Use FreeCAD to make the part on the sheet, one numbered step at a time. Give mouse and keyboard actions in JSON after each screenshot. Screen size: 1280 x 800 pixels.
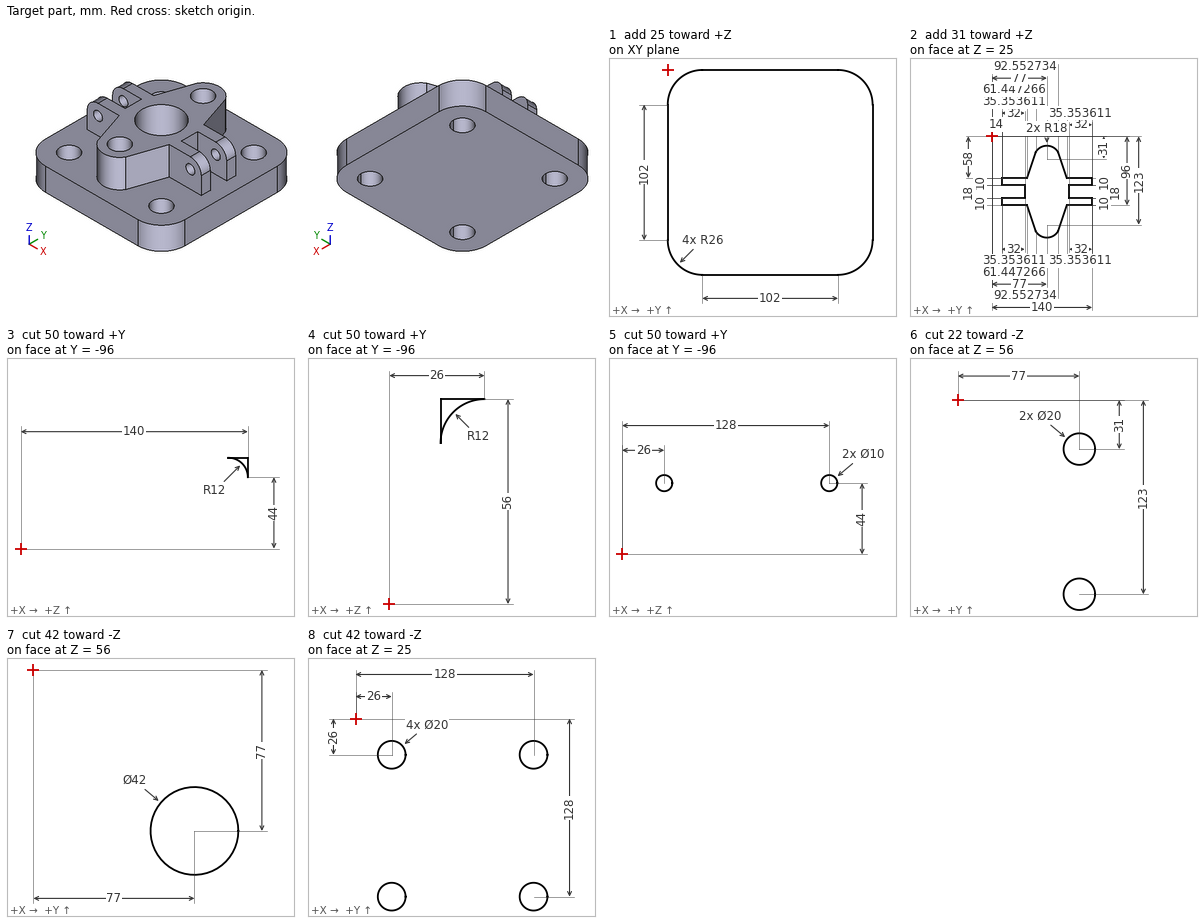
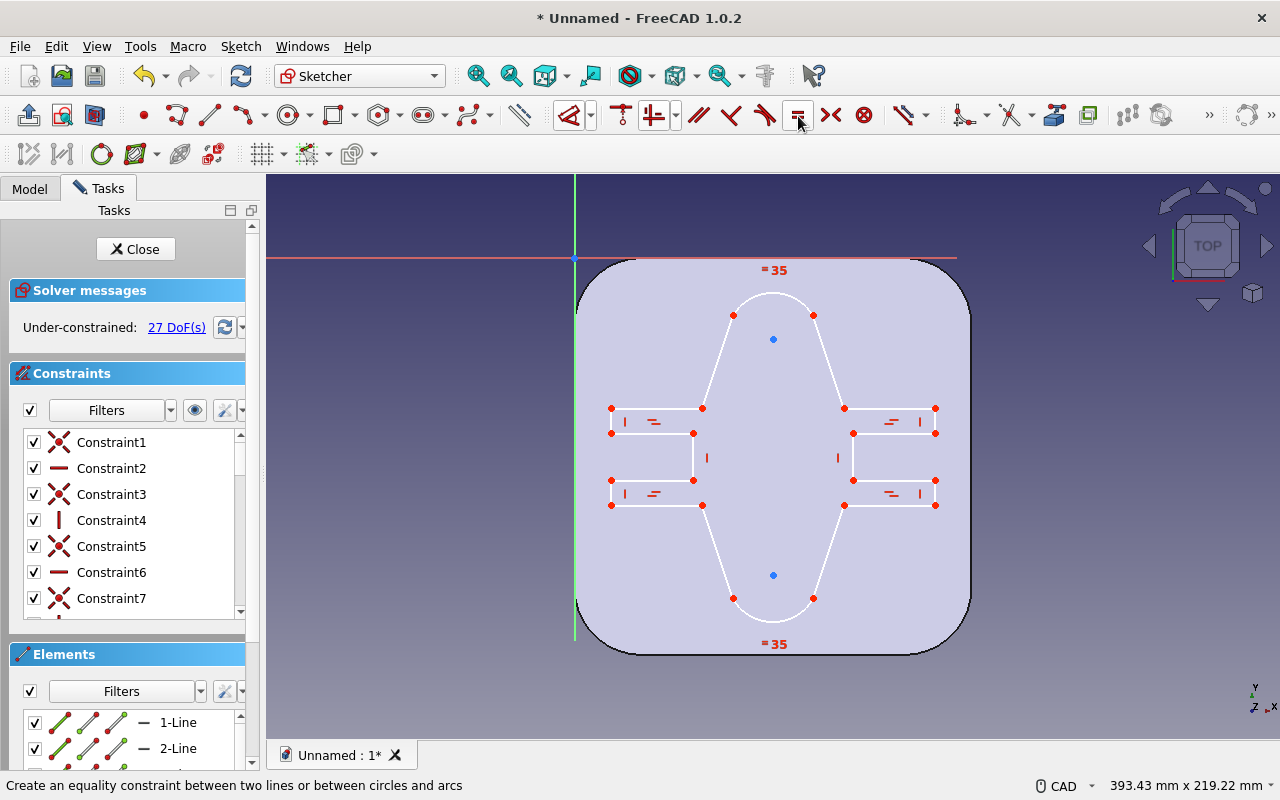
{"action": "left_click", "coordinate": [792, 297]}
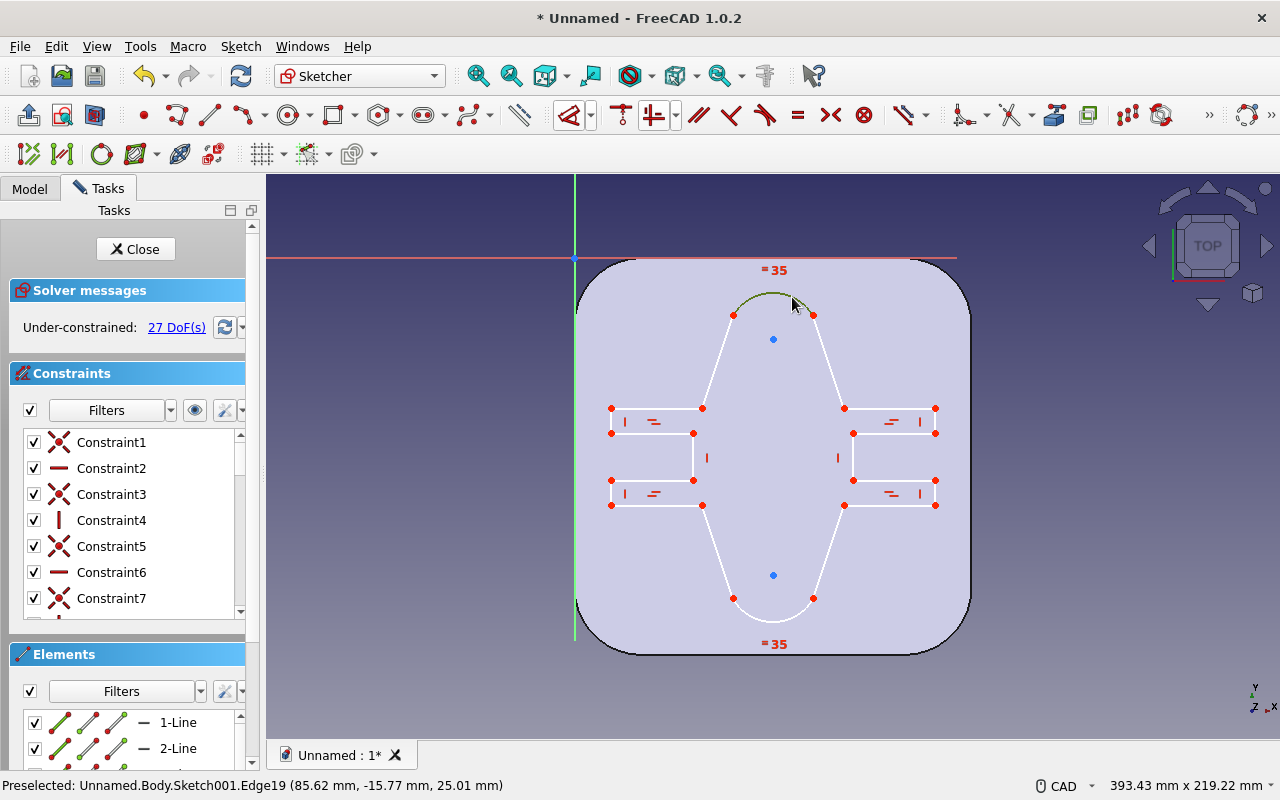
{"action": "left_click", "coordinate": [590, 116]}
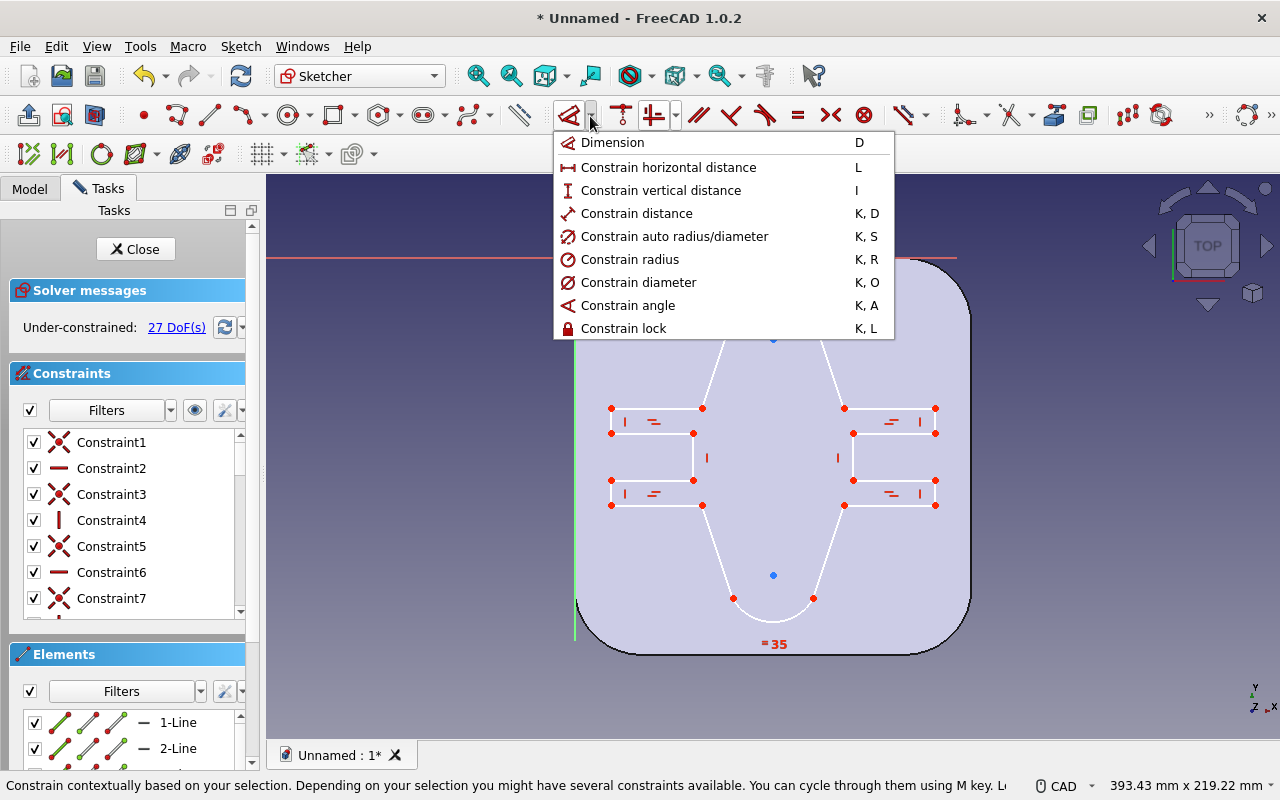
{"action": "left_click", "coordinate": [724, 260]}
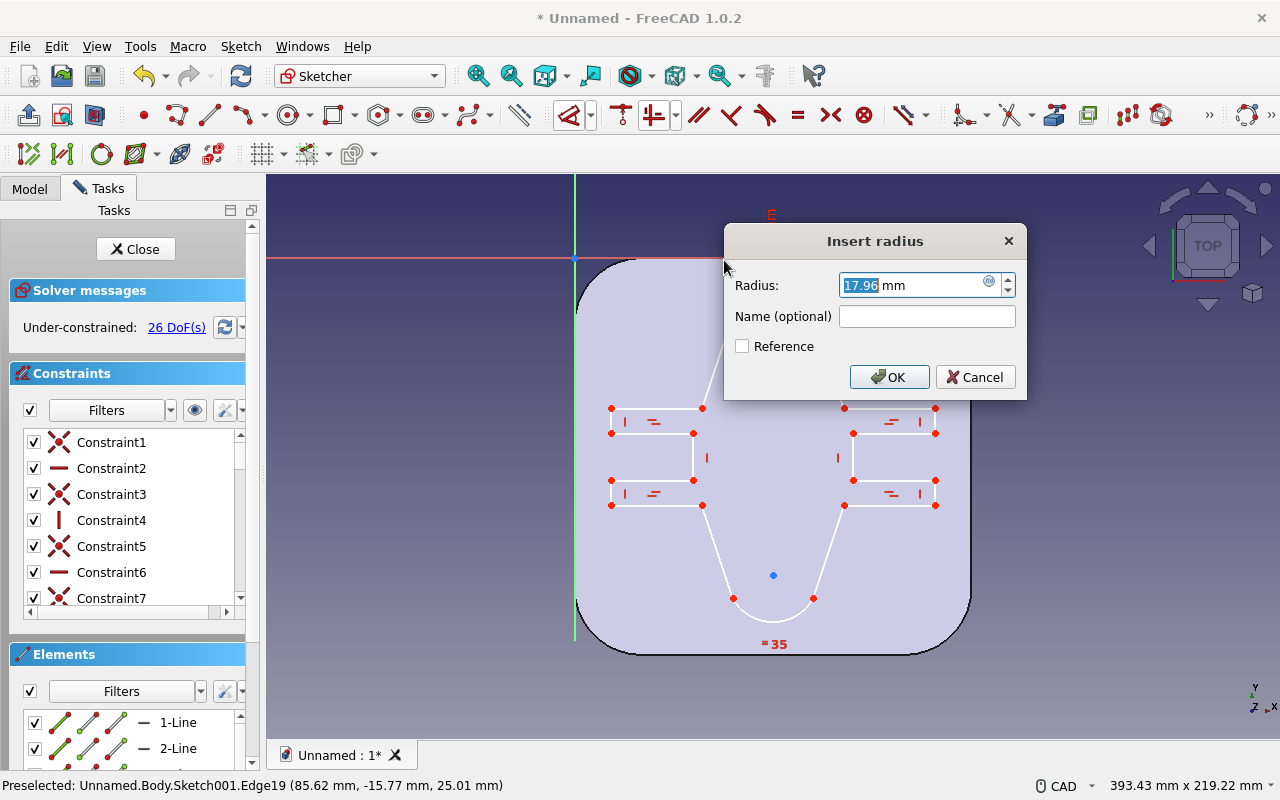
{"action": "type", "text": "18"}
{"action": "key", "text": "Return"}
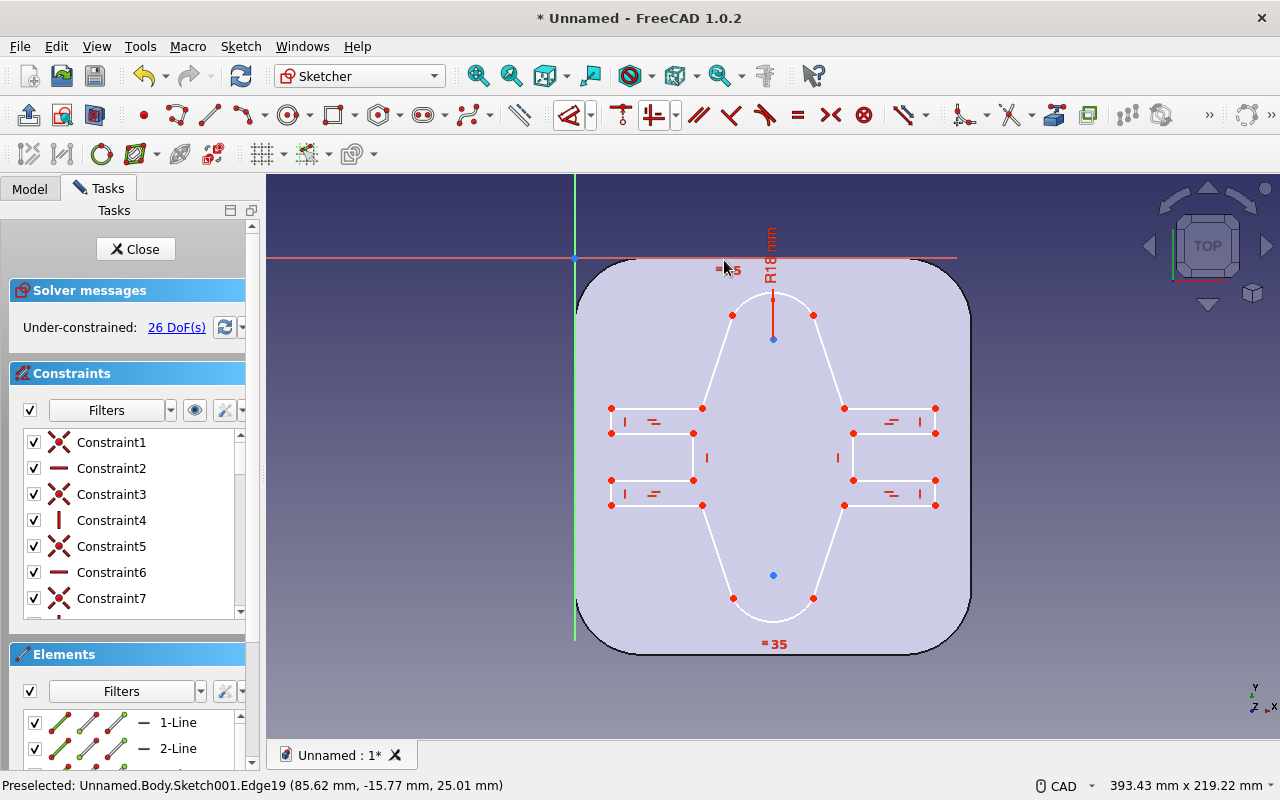
{"action": "scroll", "coordinate": [935, 496], "scroll_direction": "up", "scroll_amount": 3}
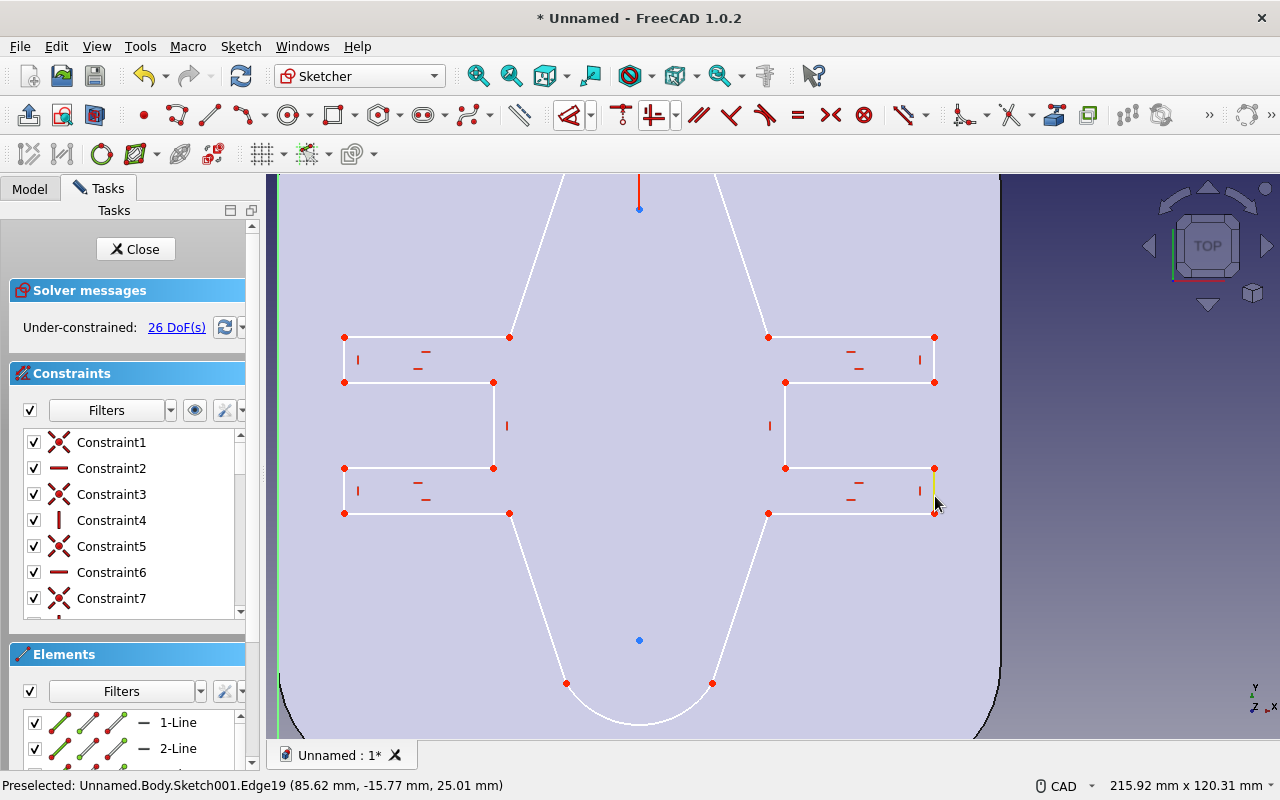
{"action": "left_click", "coordinate": [934, 496]}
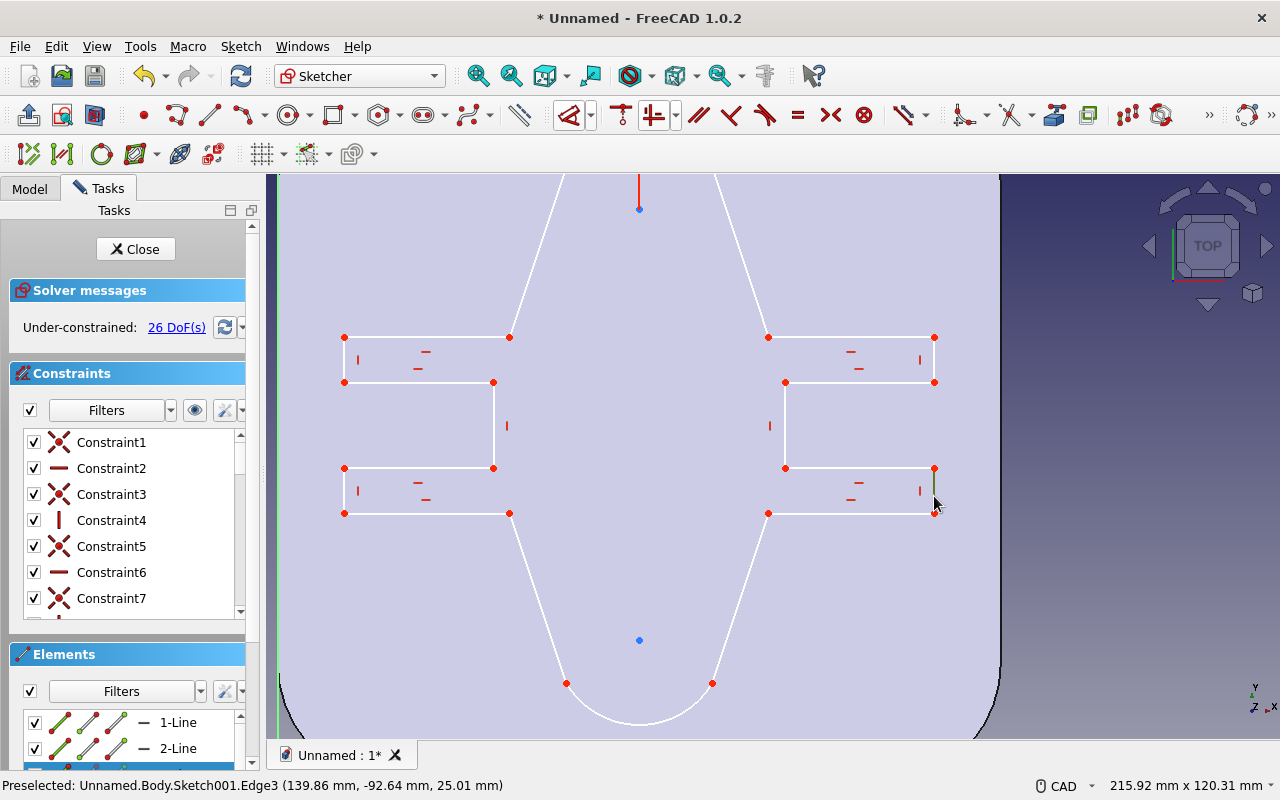
{"action": "left_click", "coordinate": [590, 116]}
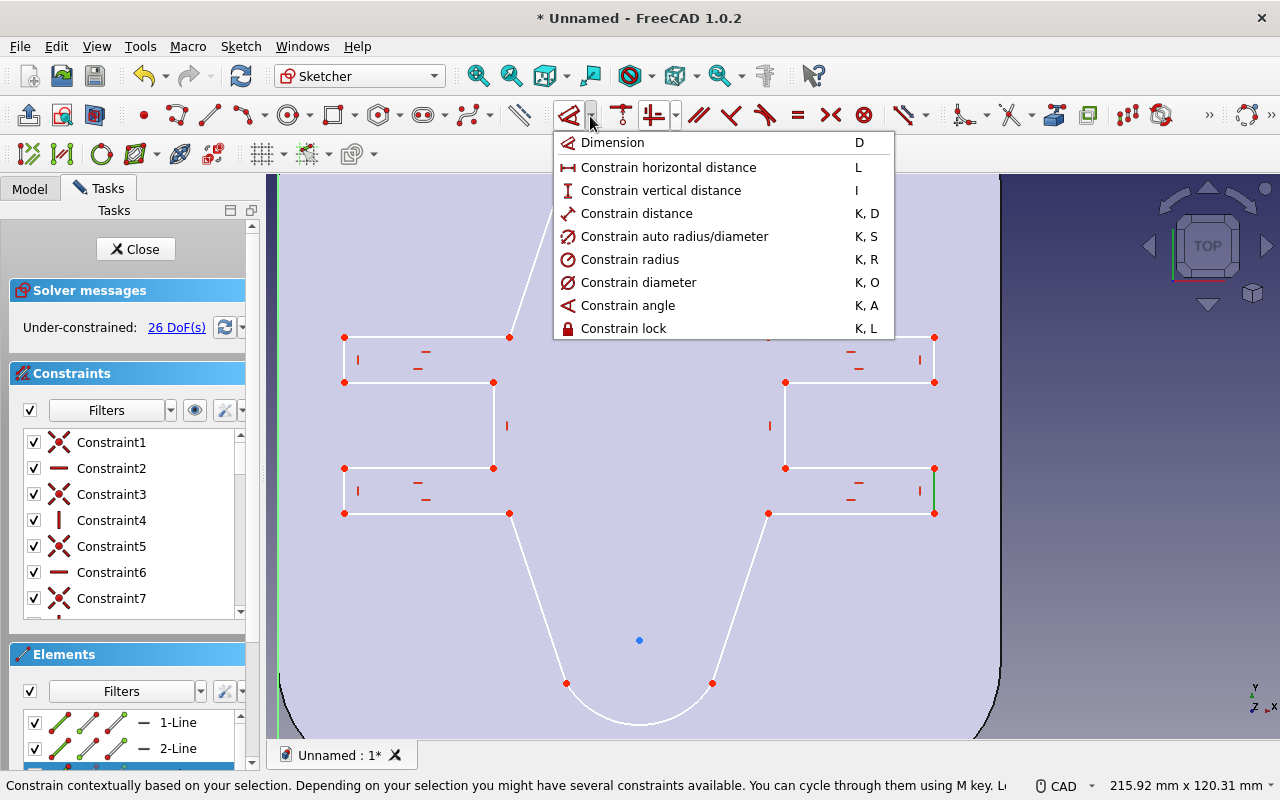
{"action": "left_click", "coordinate": [724, 190]}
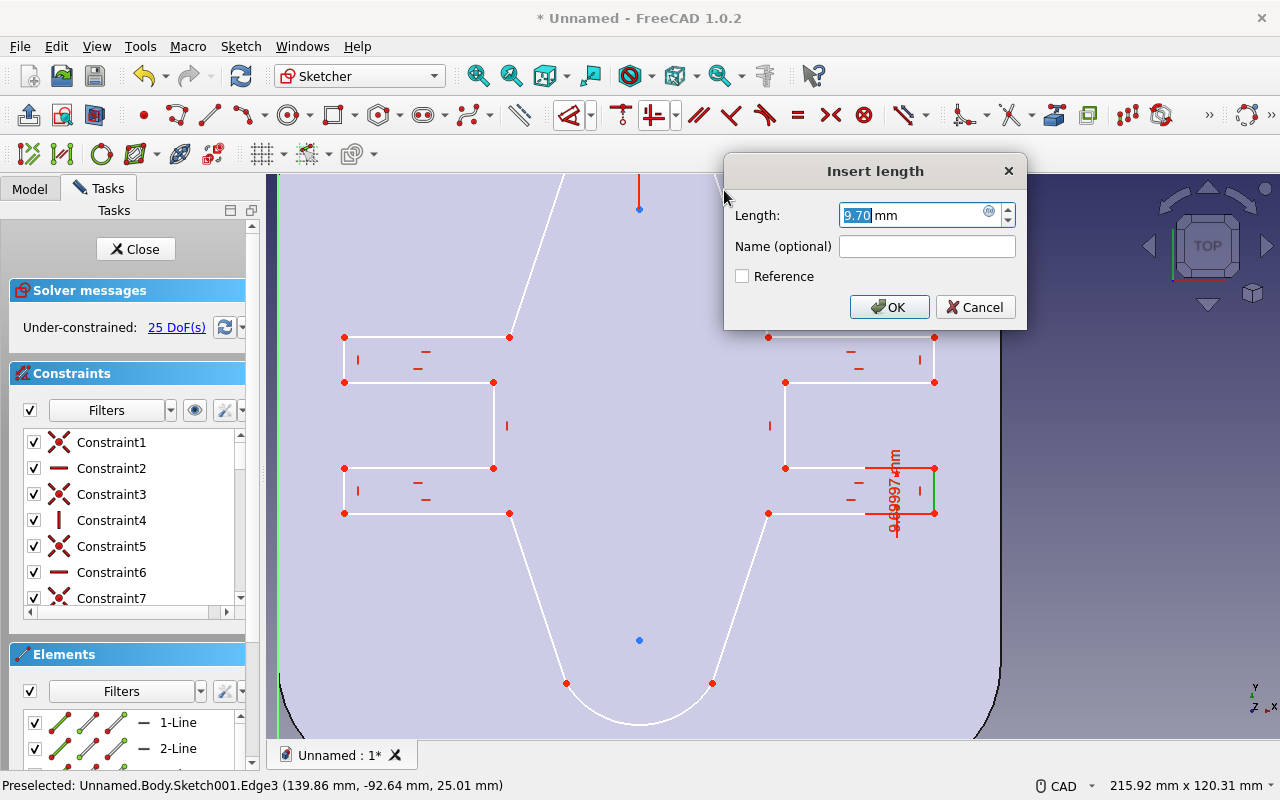
{"action": "type", "text": "10"}
{"action": "key", "text": "Return"}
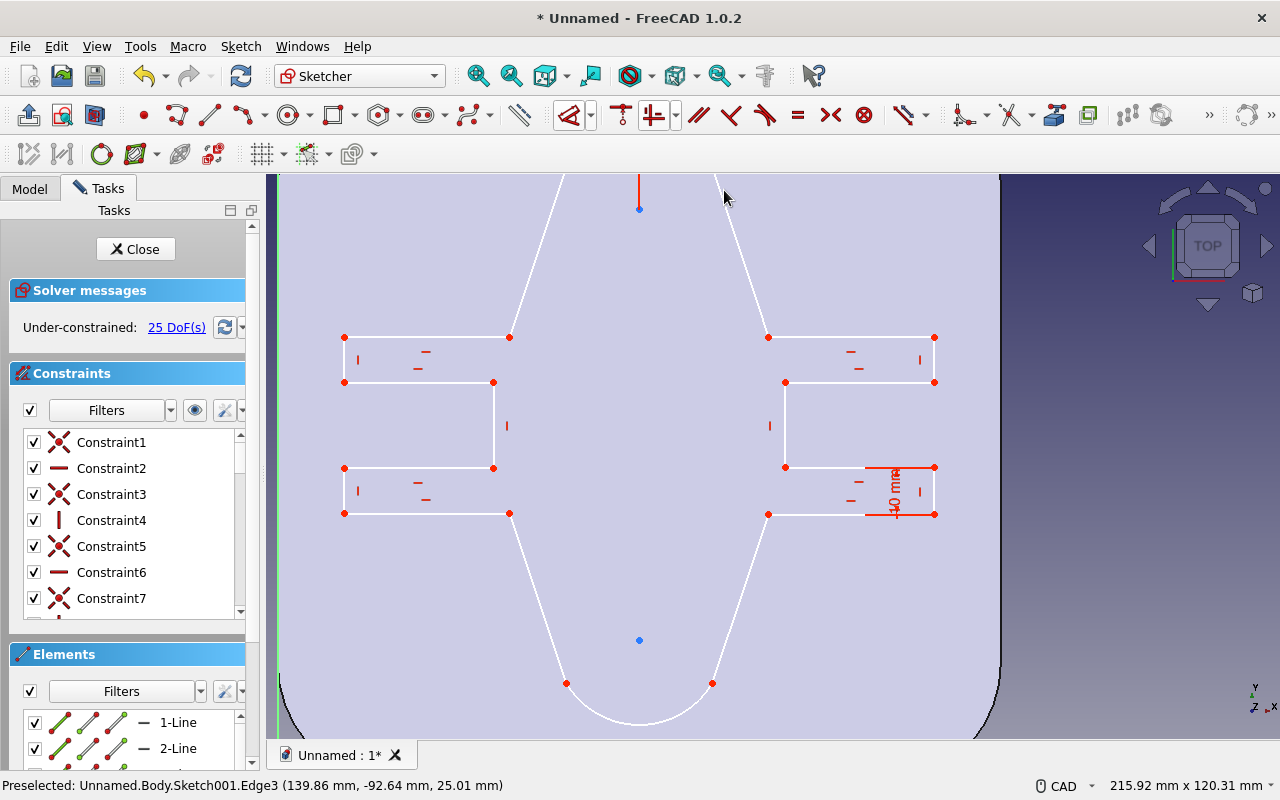
{"action": "left_click", "coordinate": [830, 468]}